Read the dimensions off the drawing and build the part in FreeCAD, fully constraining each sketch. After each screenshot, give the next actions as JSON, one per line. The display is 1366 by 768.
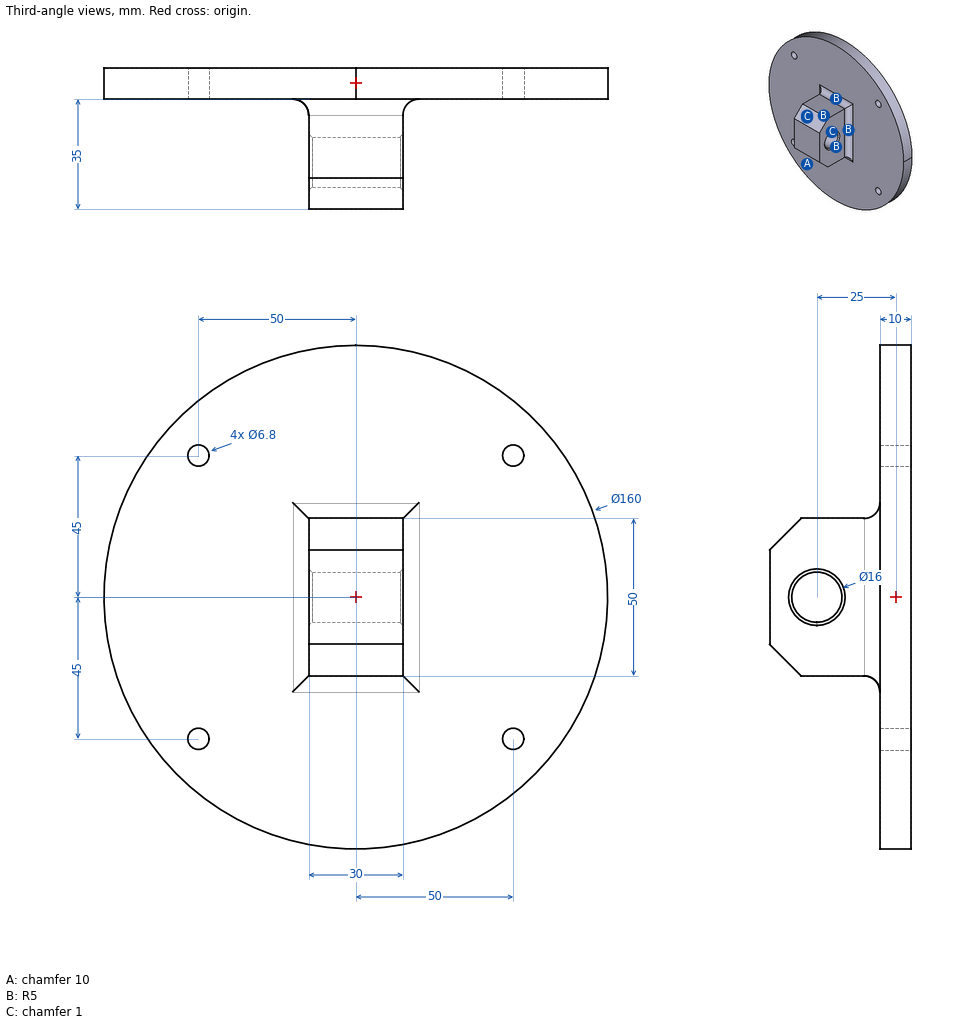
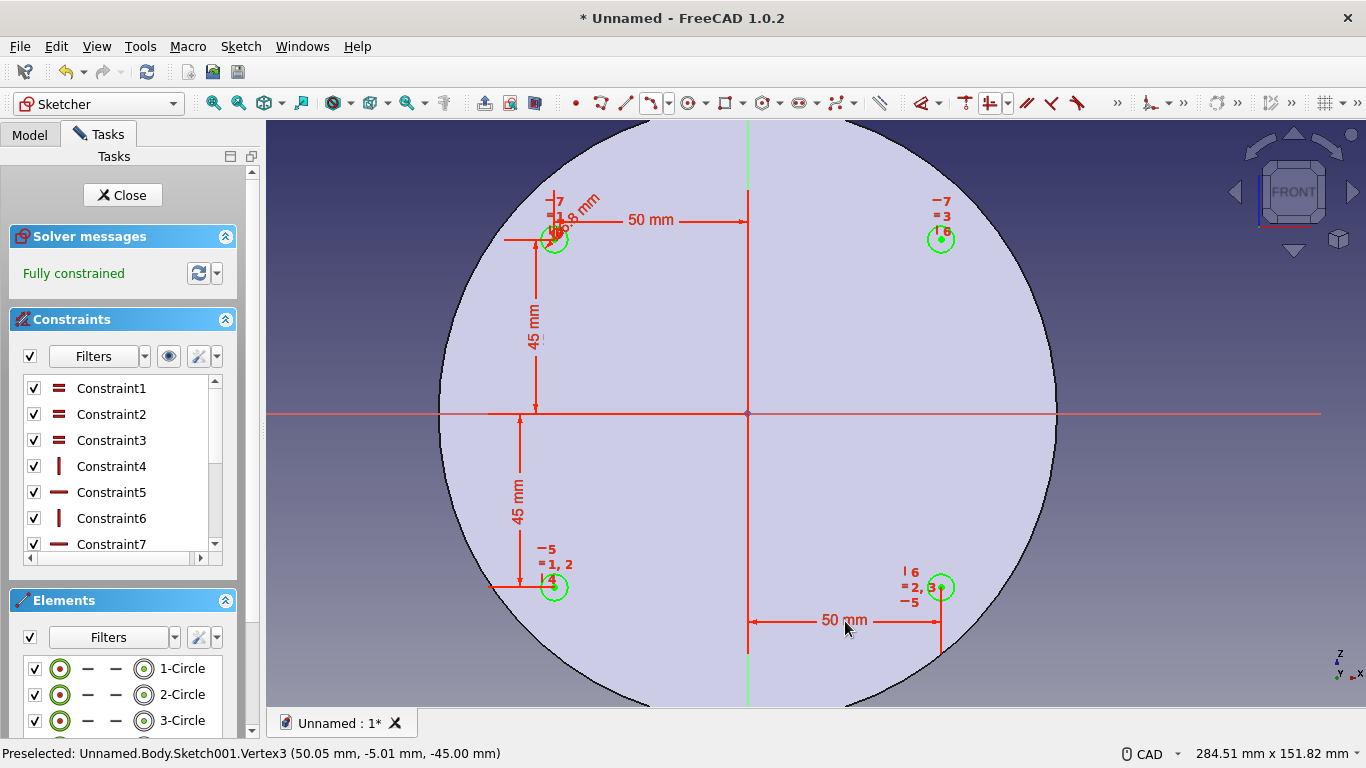
{"action": "left_click", "coordinate": [123, 195]}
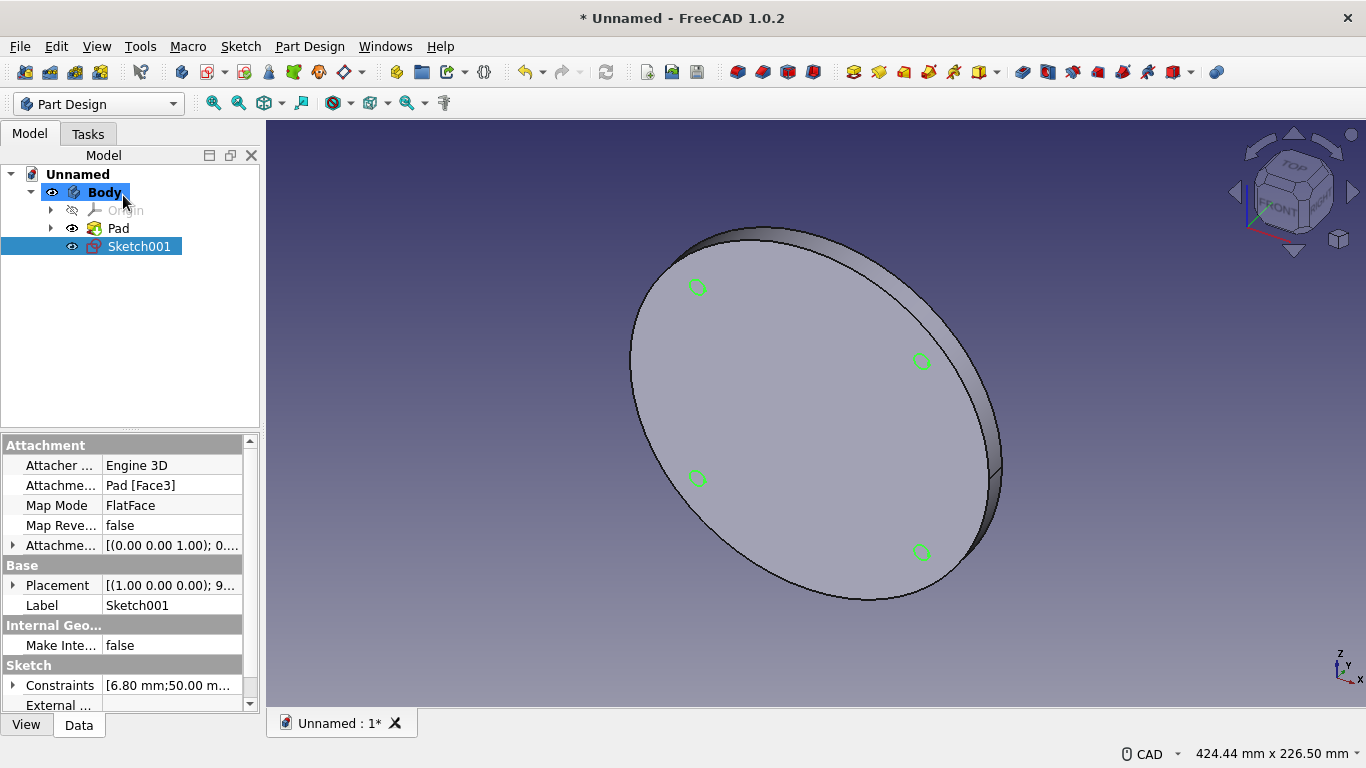
{"action": "left_click", "coordinate": [1023, 72]}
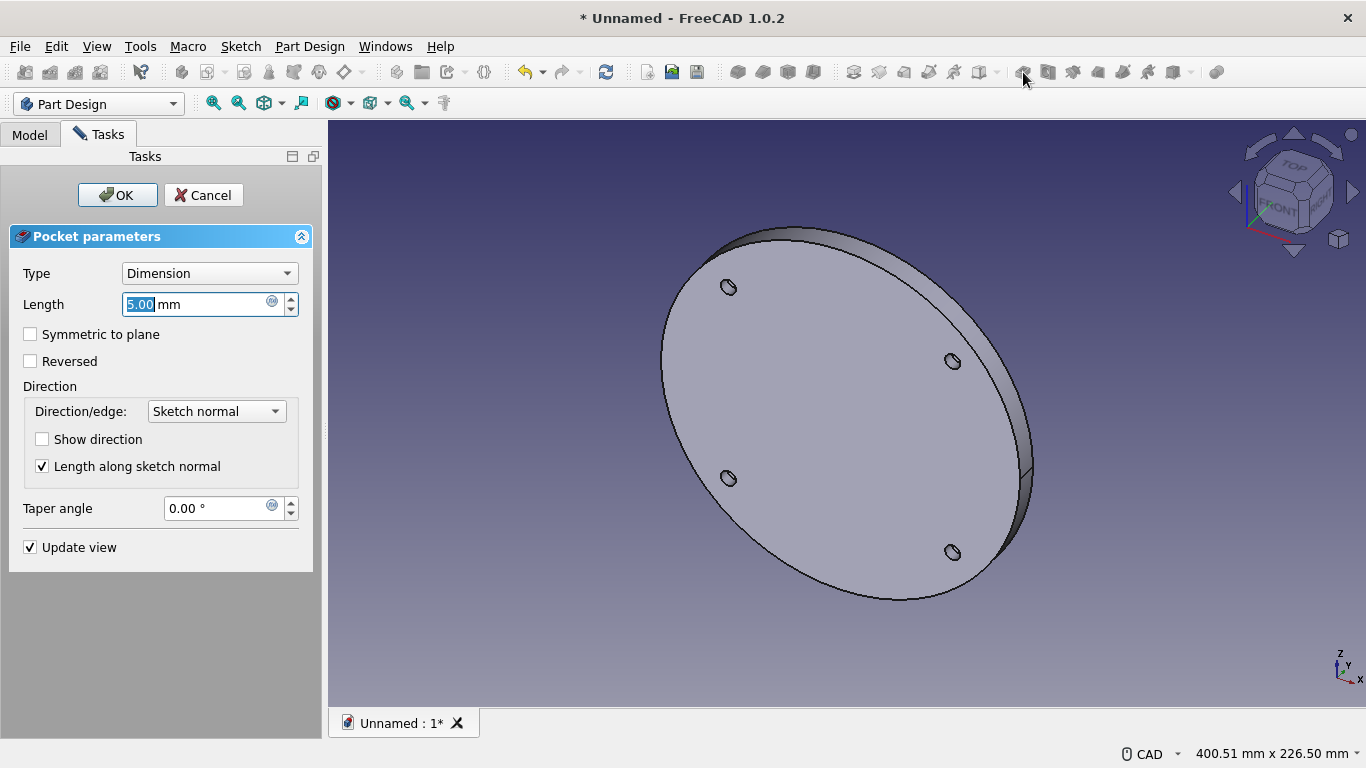
{"action": "left_click", "coordinate": [210, 274]}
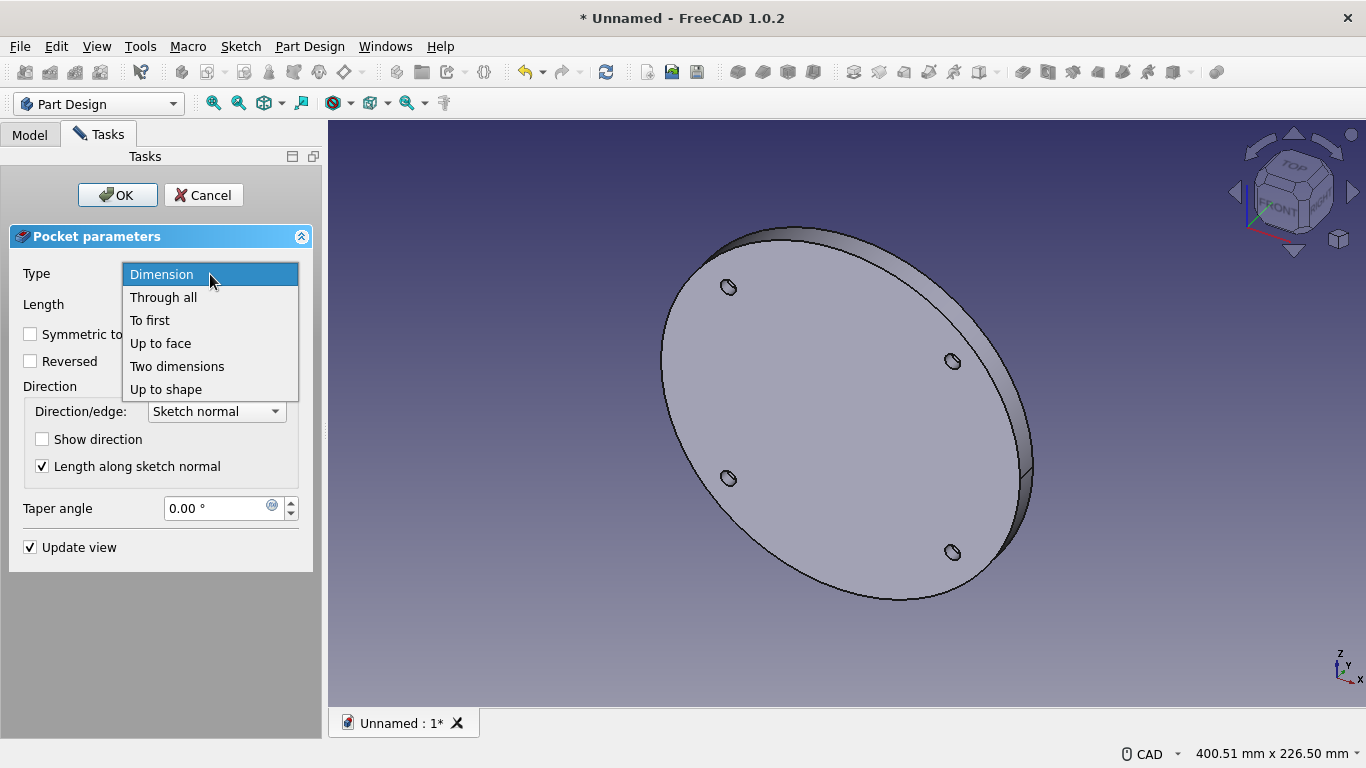
{"action": "left_click", "coordinate": [208, 298]}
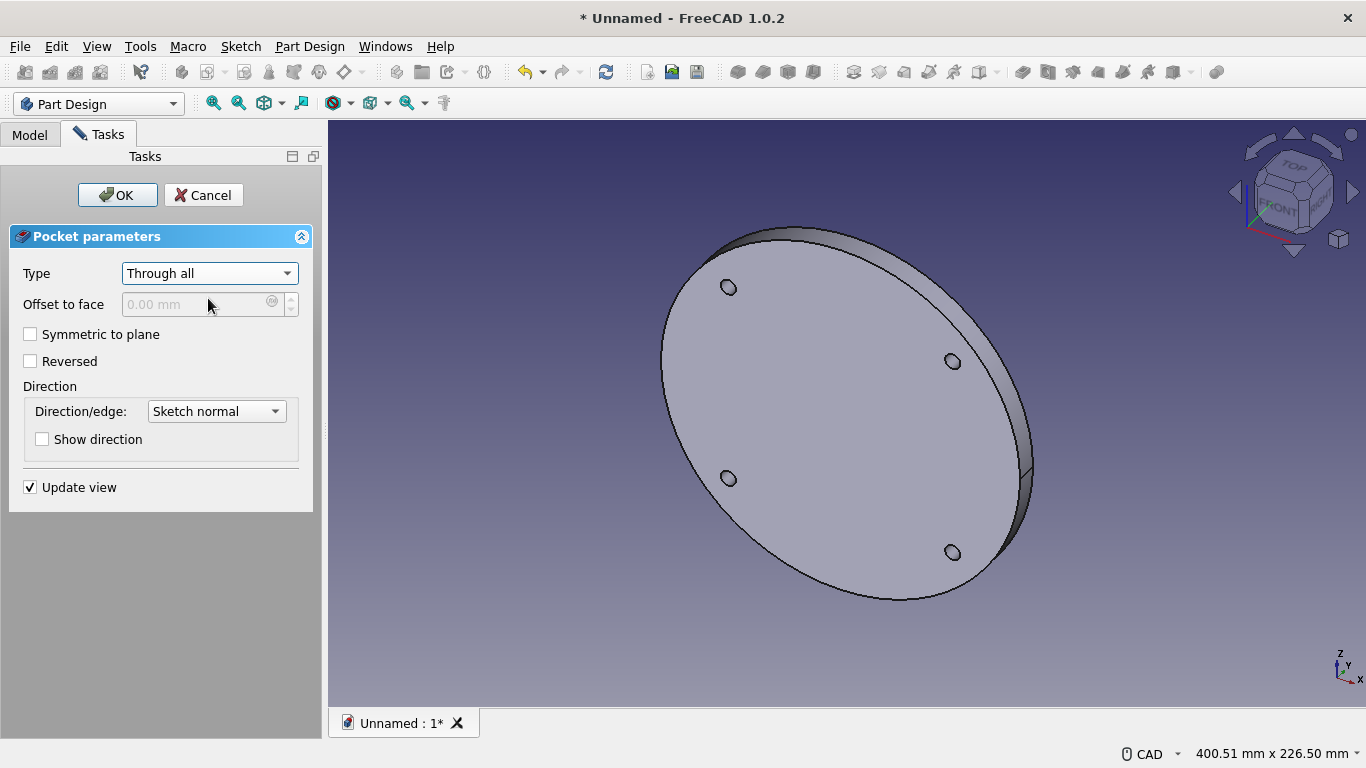
{"action": "left_click", "coordinate": [118, 195]}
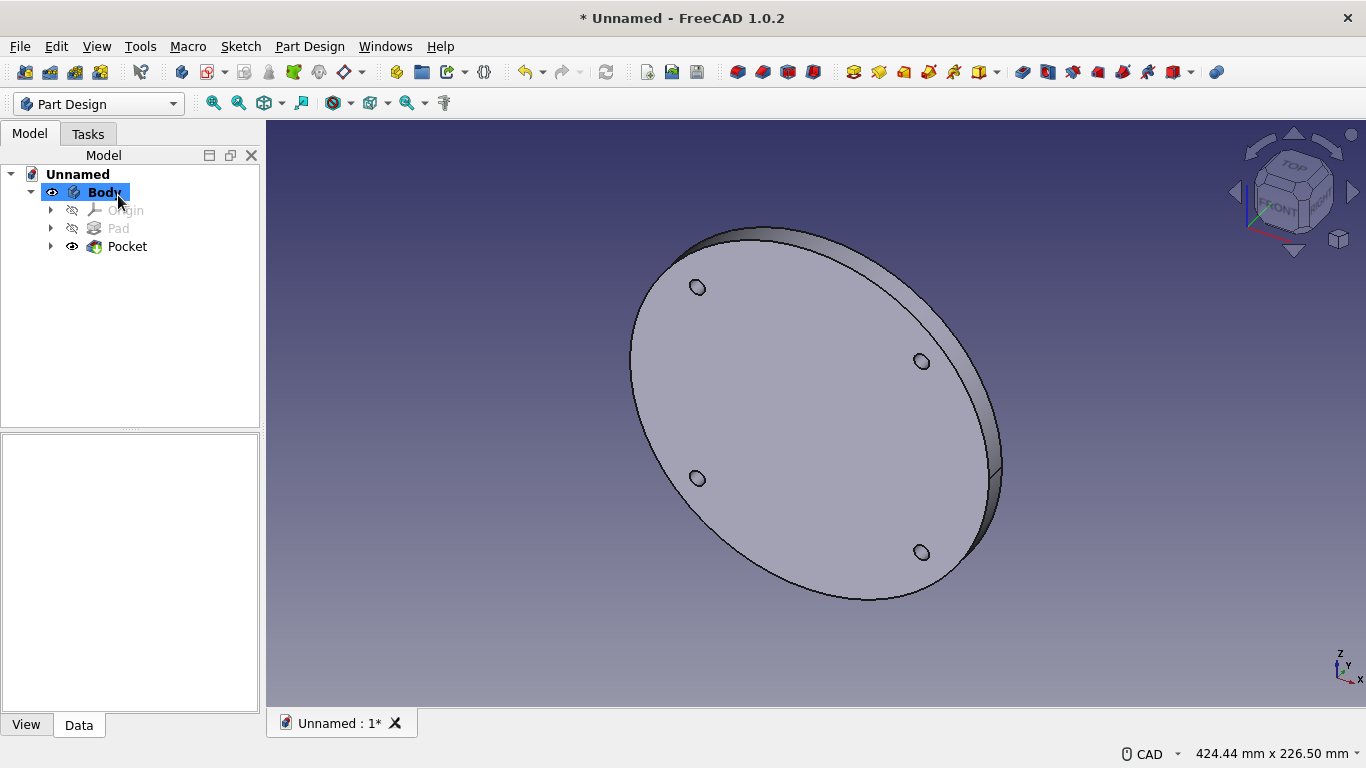
{"action": "left_click", "coordinate": [810, 419]}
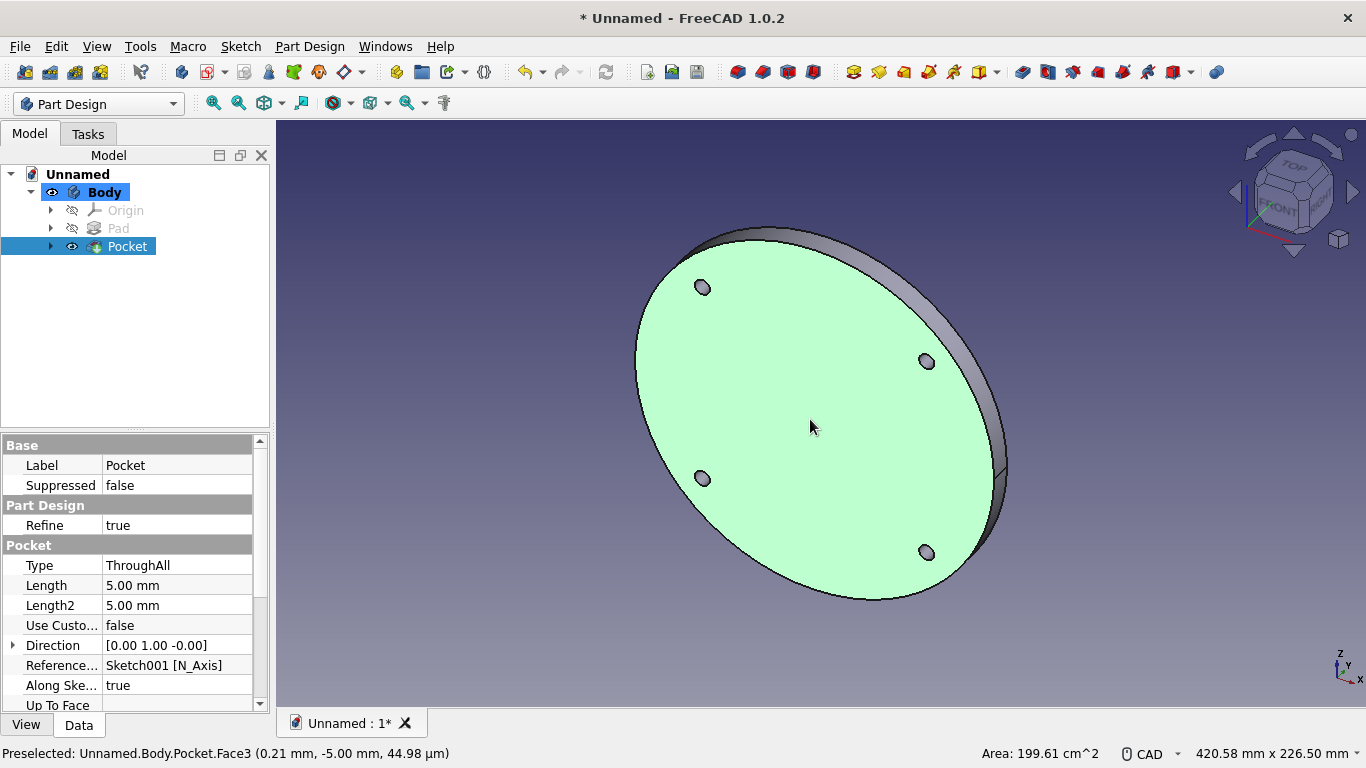
{"action": "left_click", "coordinate": [206, 72]}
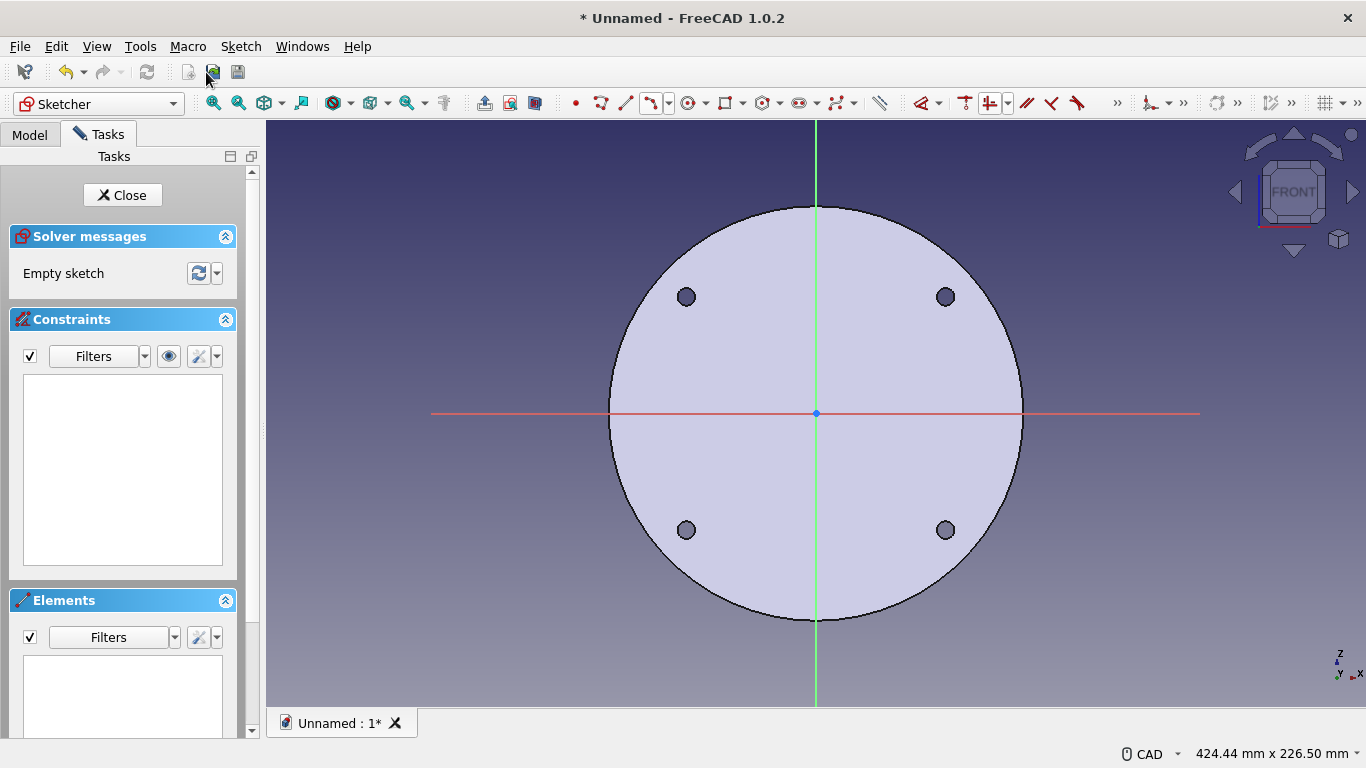
{"action": "scroll", "coordinate": [856, 414], "scroll_direction": "up", "scroll_amount": 5}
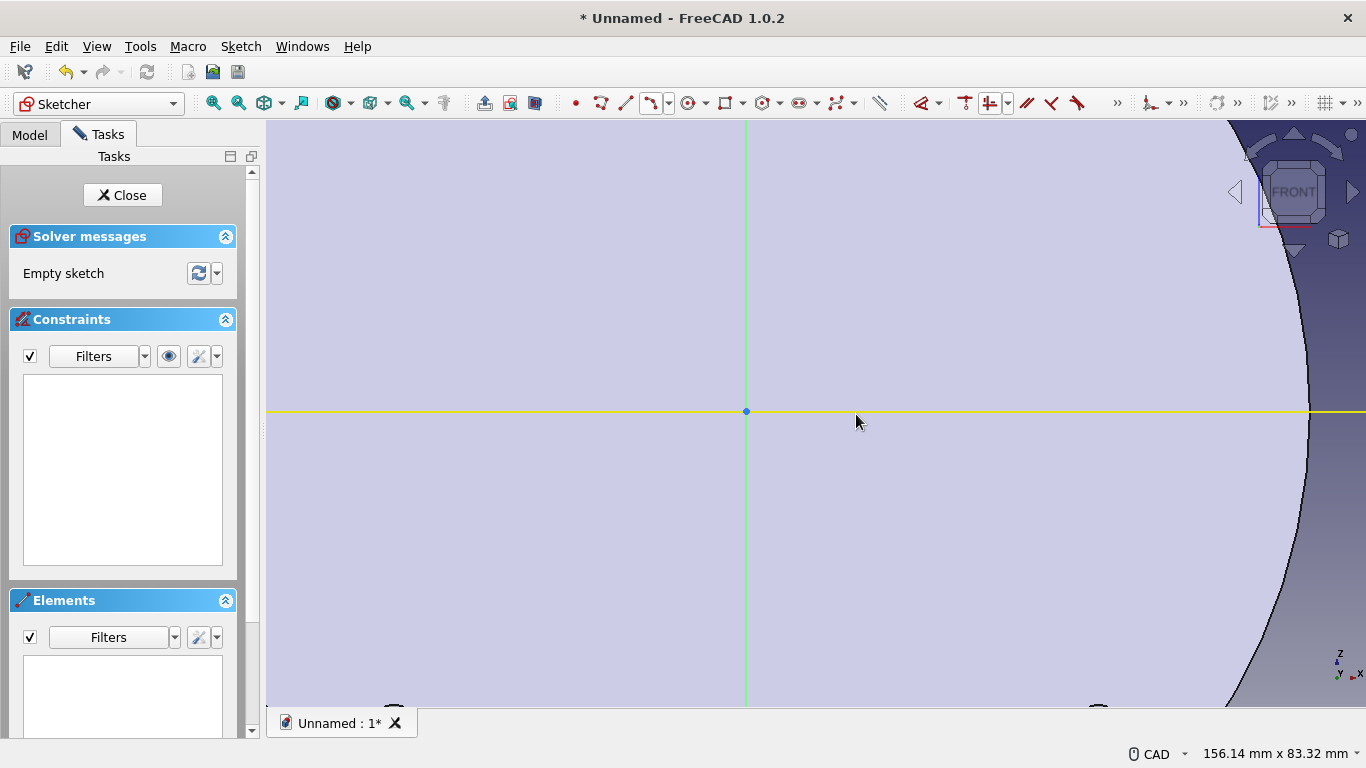
{"action": "key", "text": "g v"}